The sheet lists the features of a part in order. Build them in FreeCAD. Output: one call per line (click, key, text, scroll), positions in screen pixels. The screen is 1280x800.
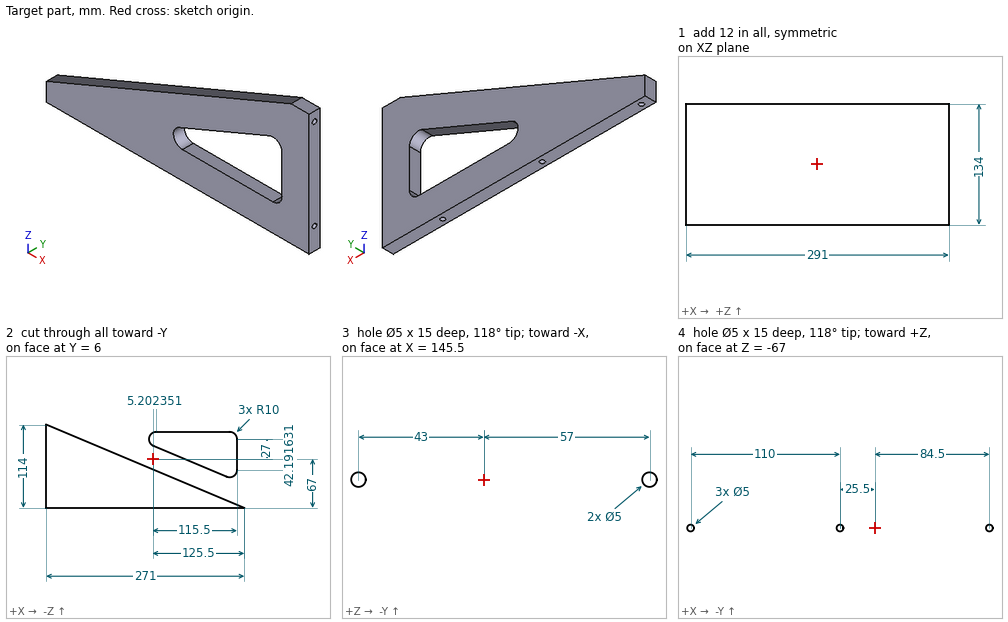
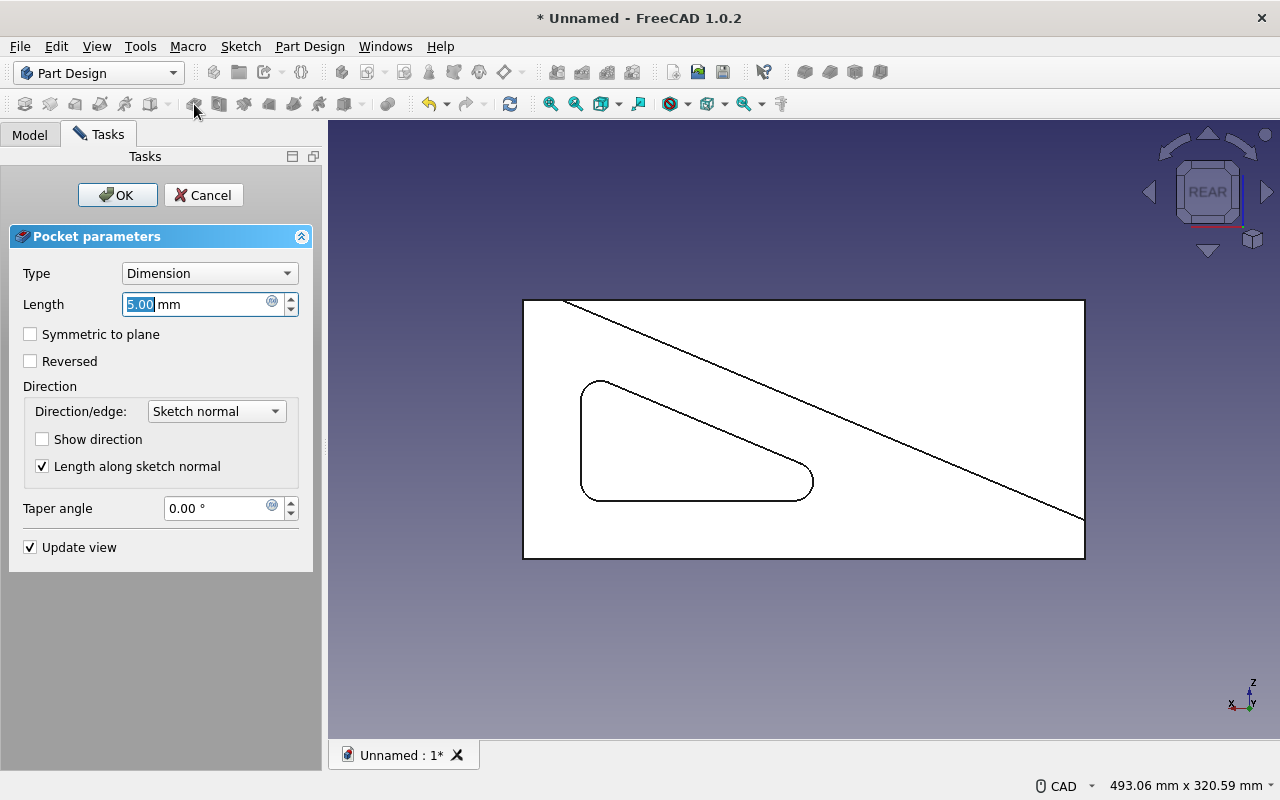
click(210, 274)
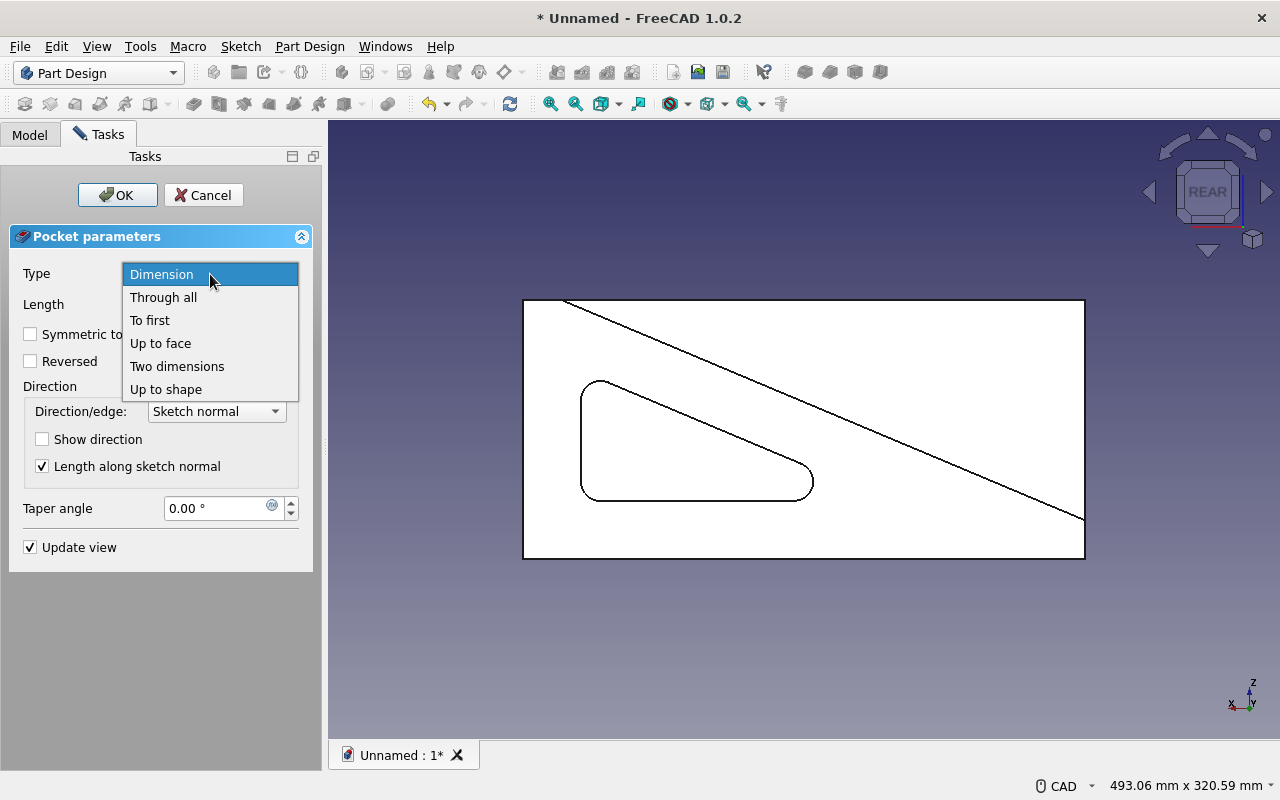
click(208, 298)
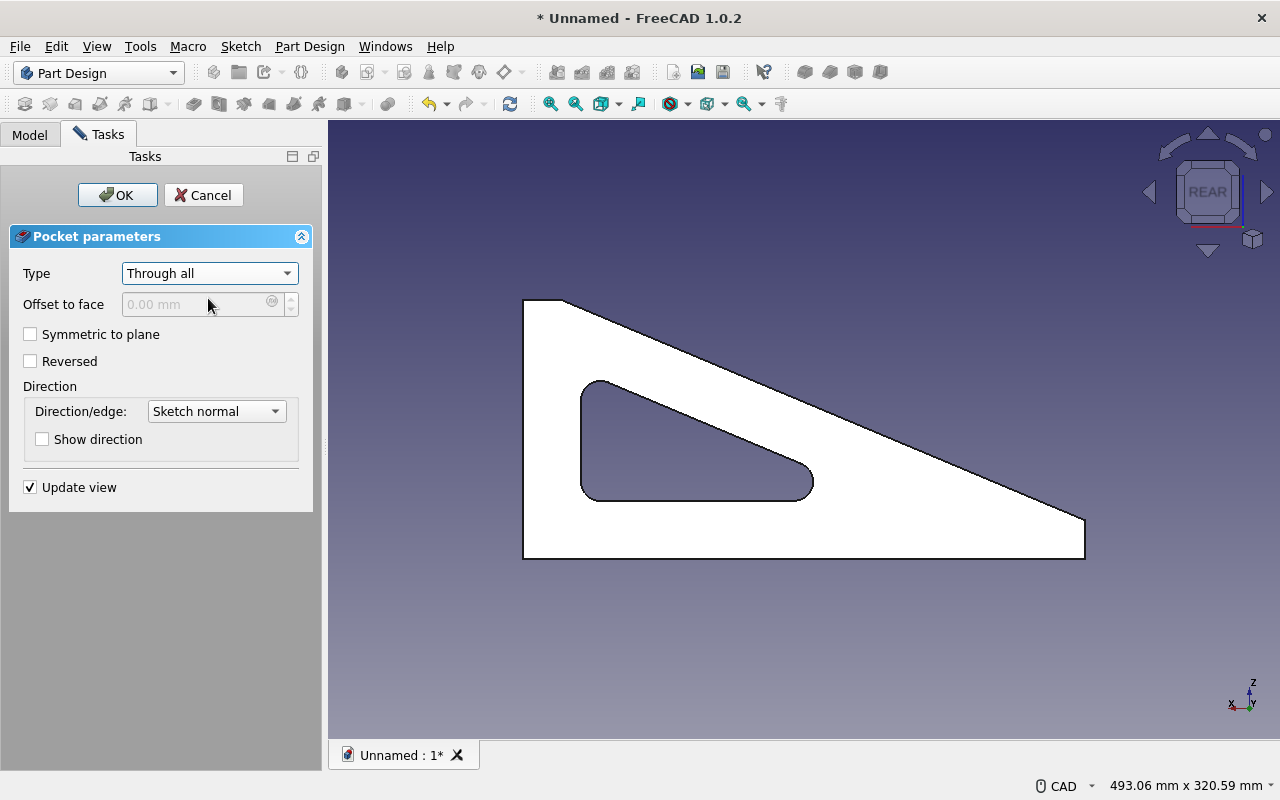
click(118, 195)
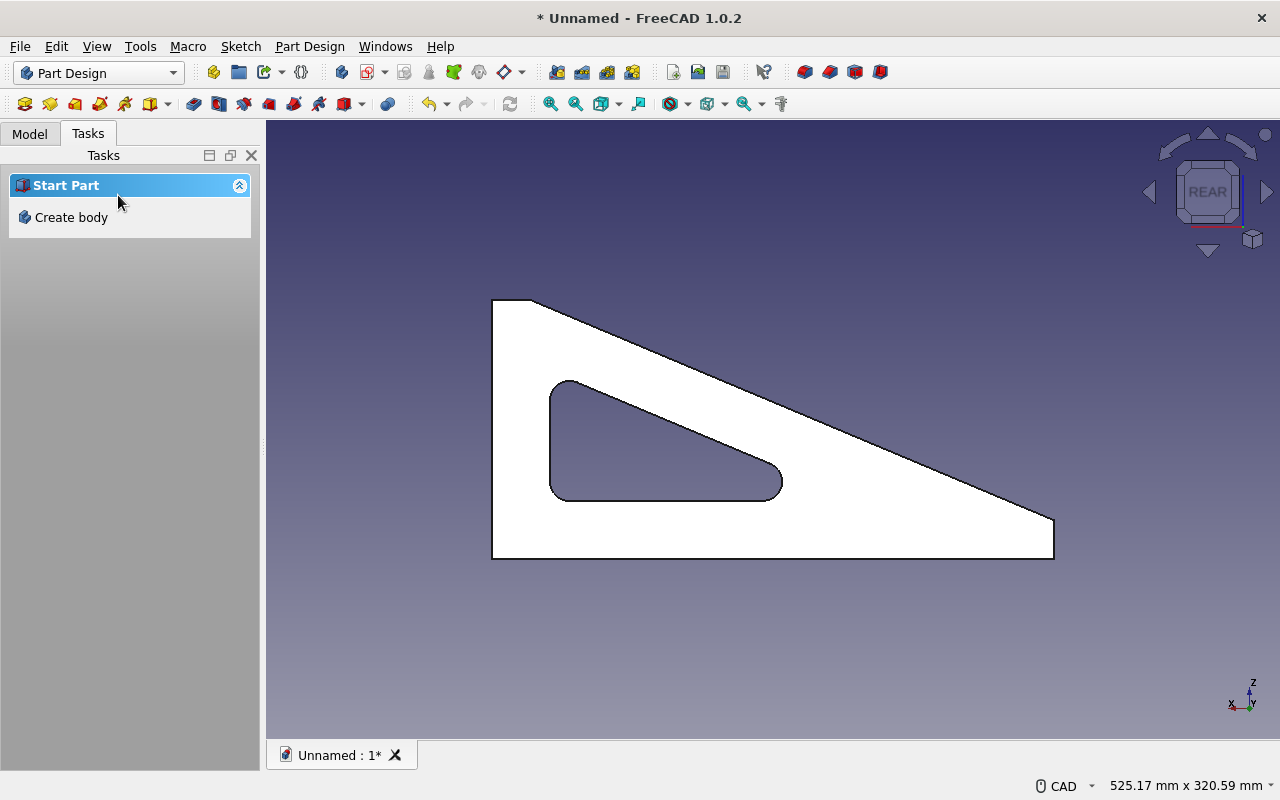
key(0)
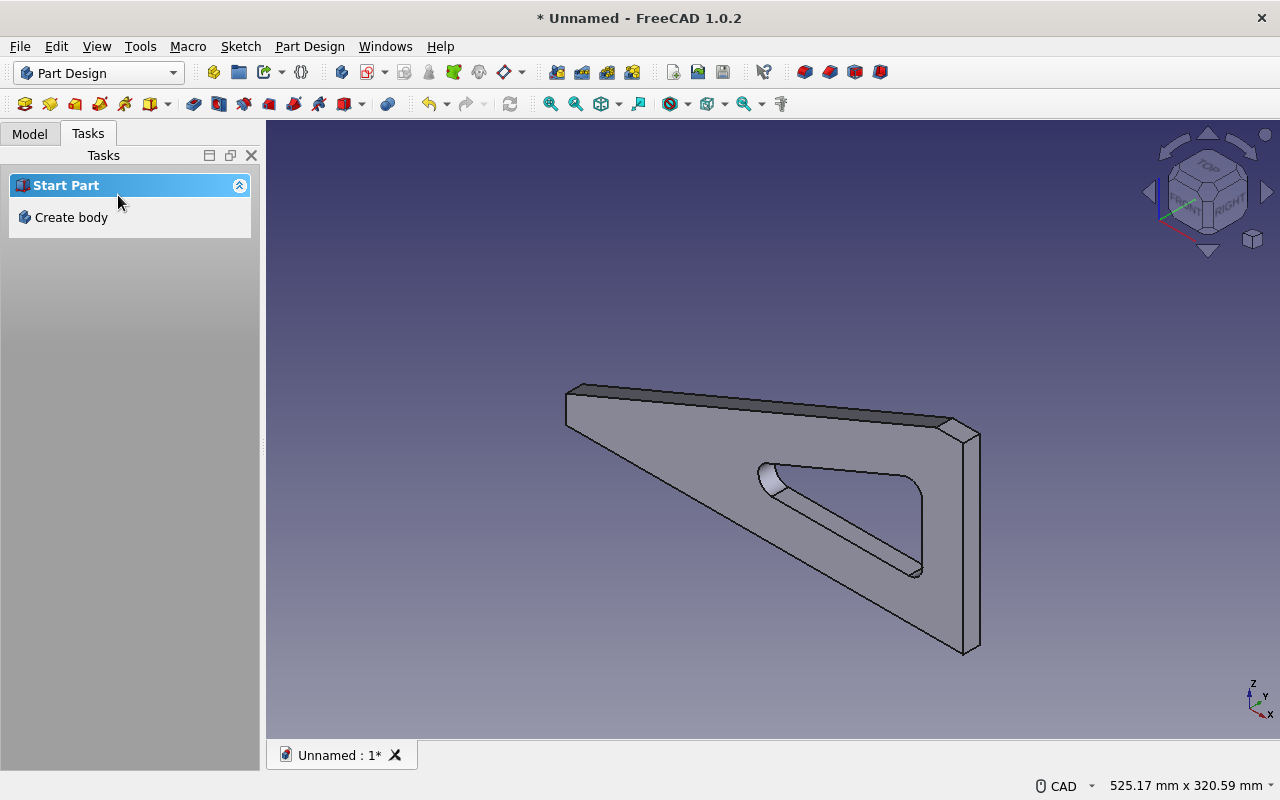
click(972, 453)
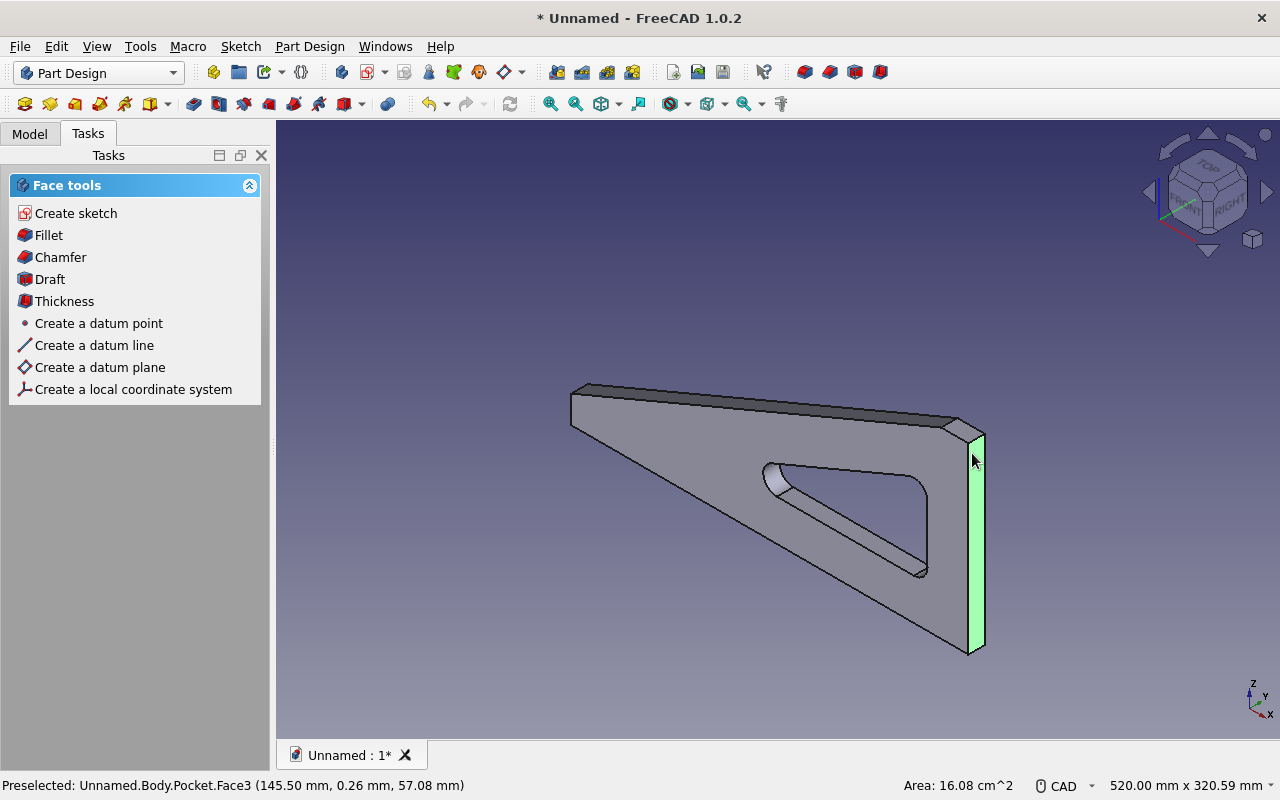
click(366, 72)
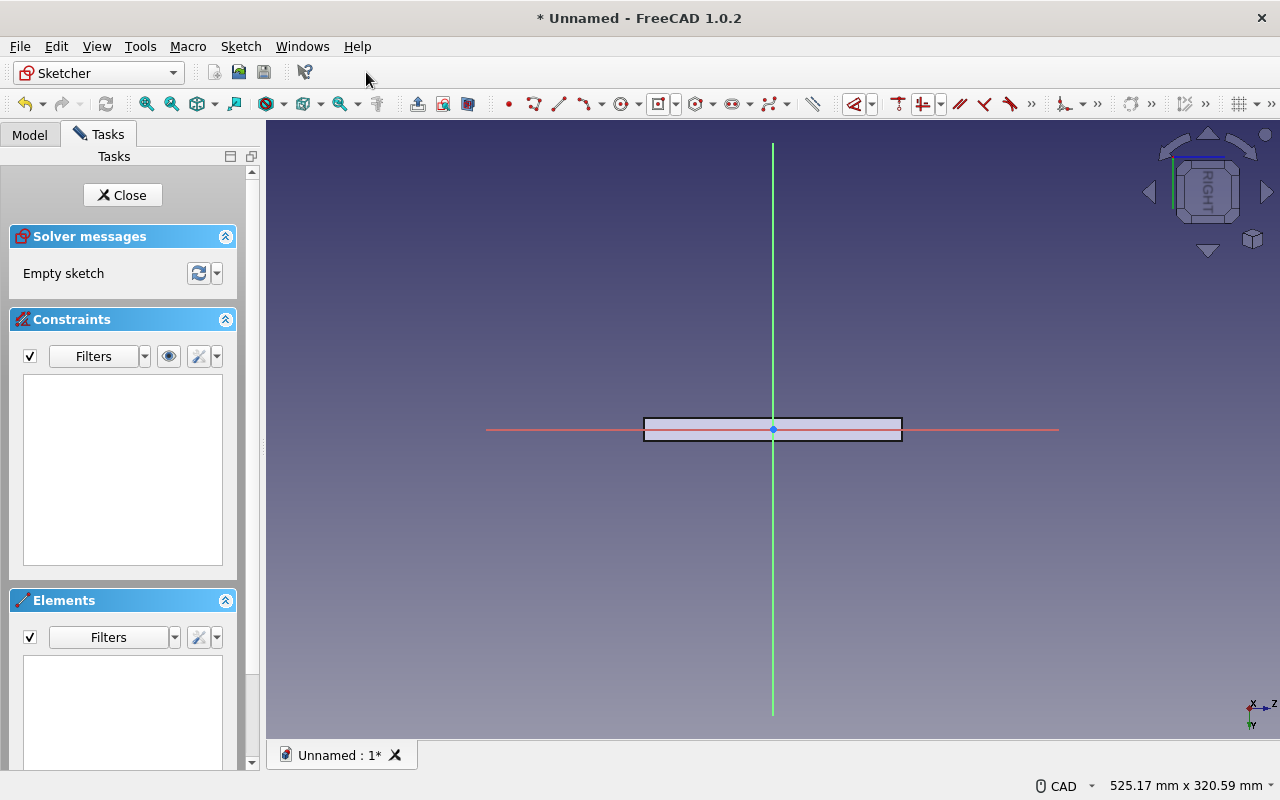
scroll(834, 430, up, 5)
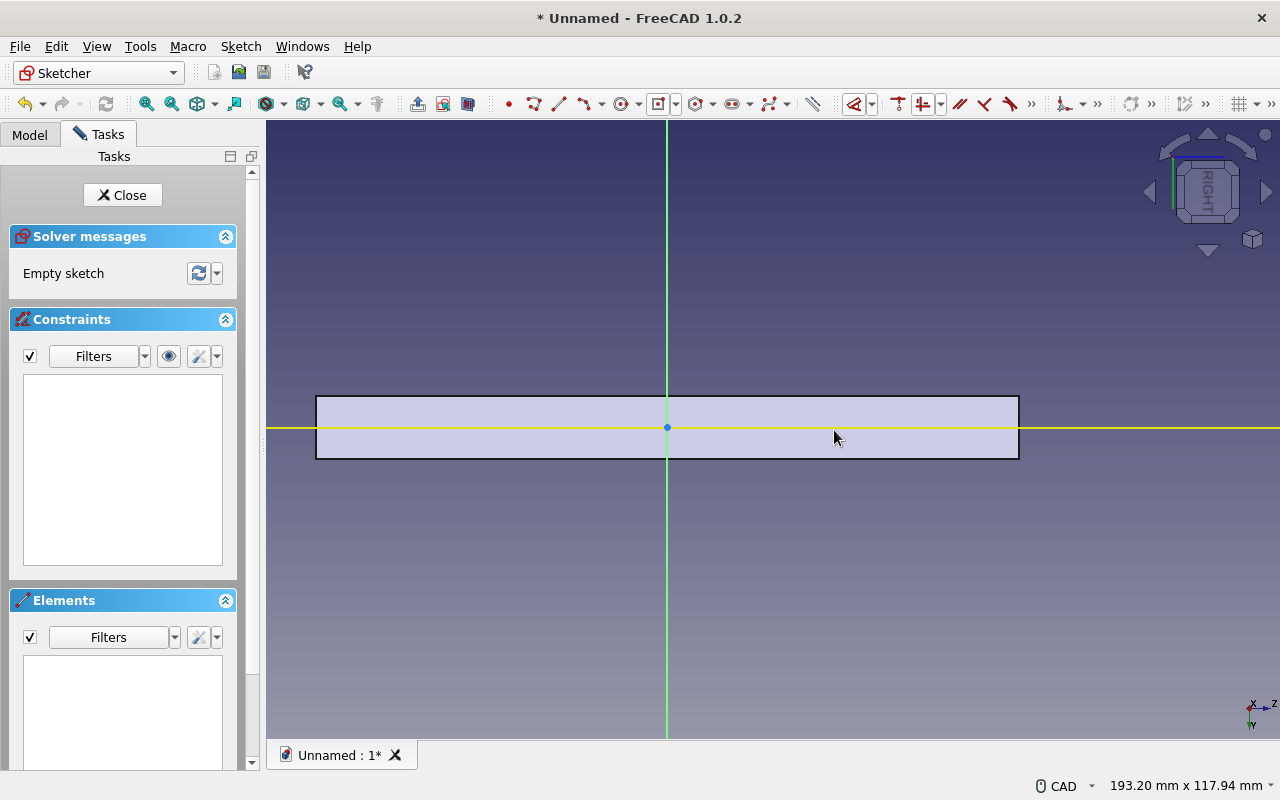
key(g)
key(c)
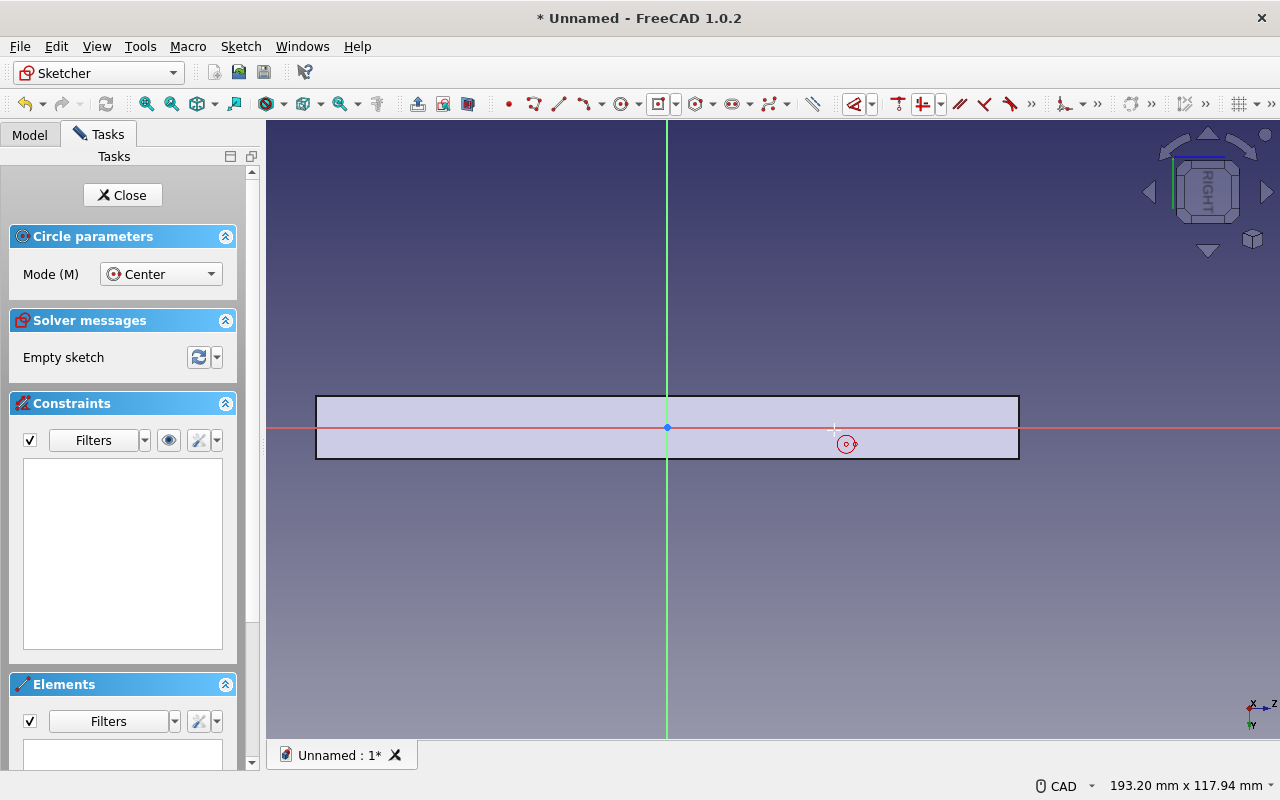
scroll(966, 428, up, 3)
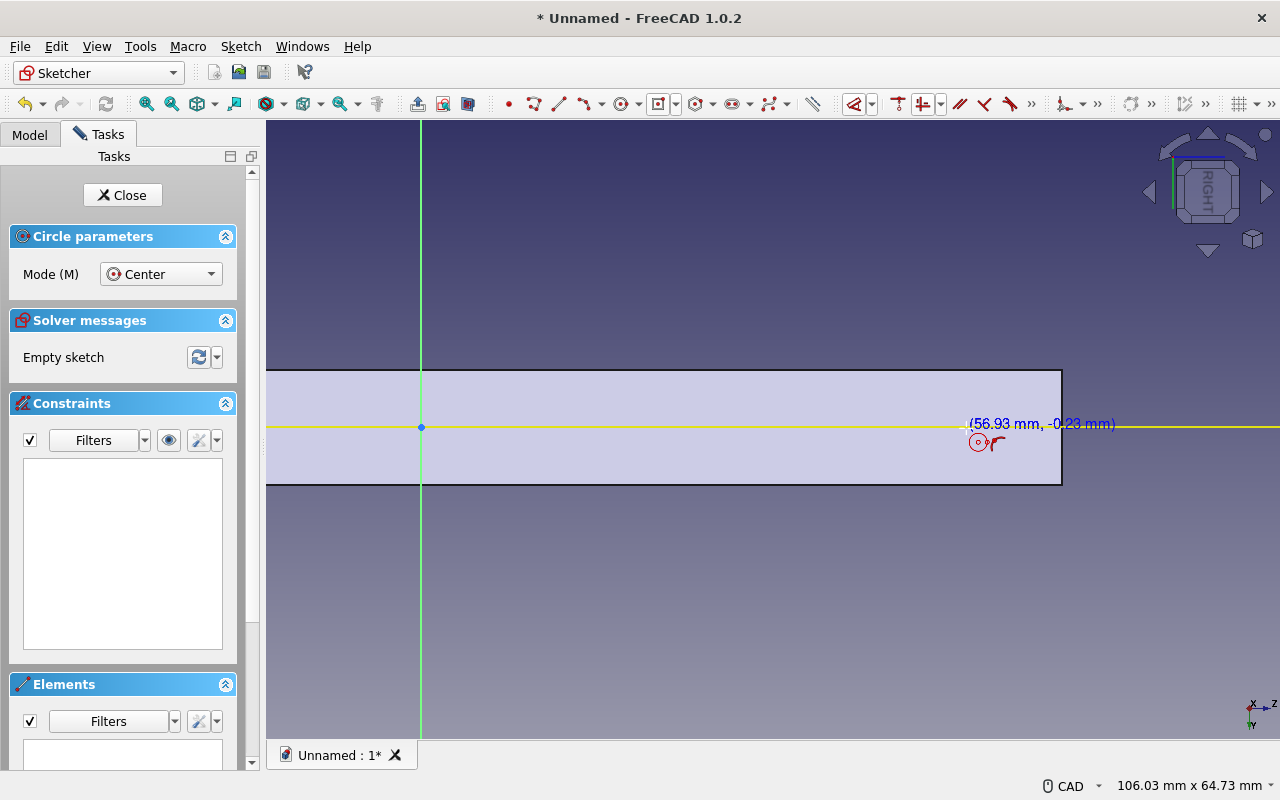
click(966, 427)
move(983, 410)